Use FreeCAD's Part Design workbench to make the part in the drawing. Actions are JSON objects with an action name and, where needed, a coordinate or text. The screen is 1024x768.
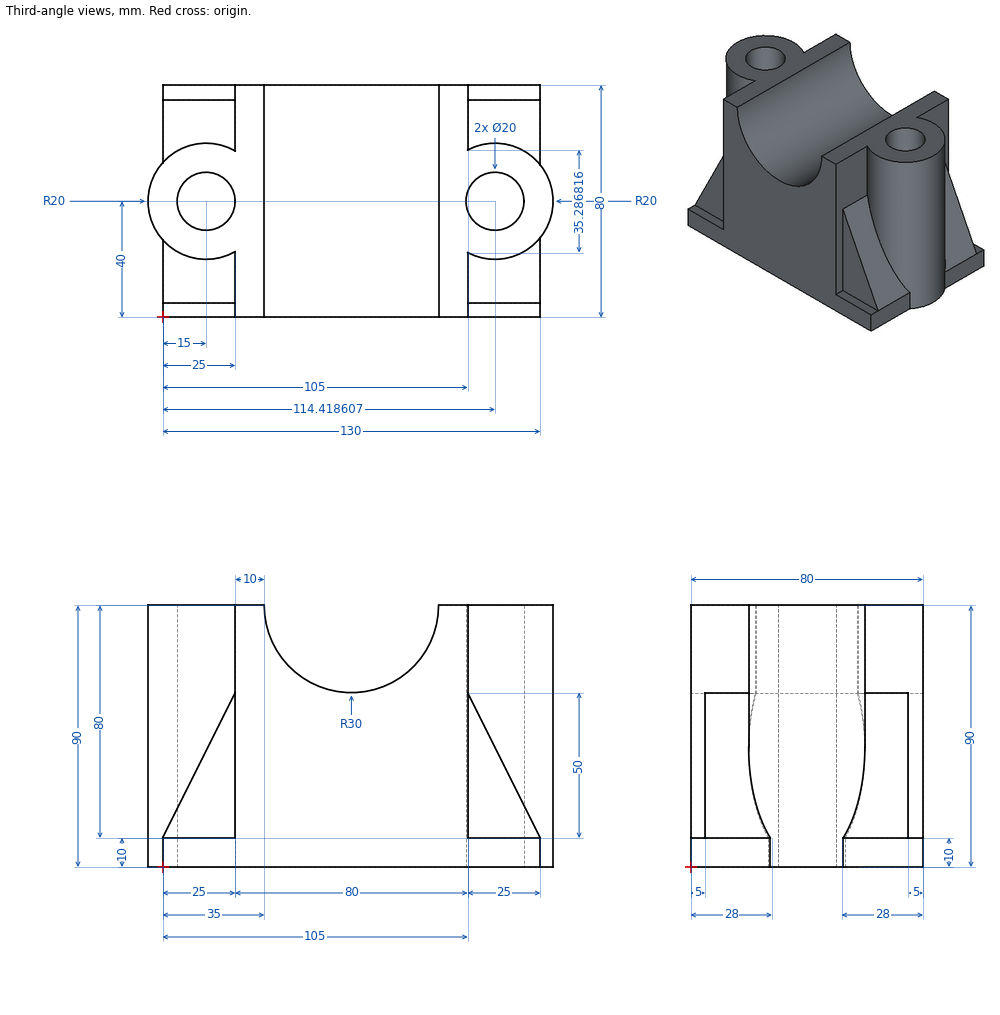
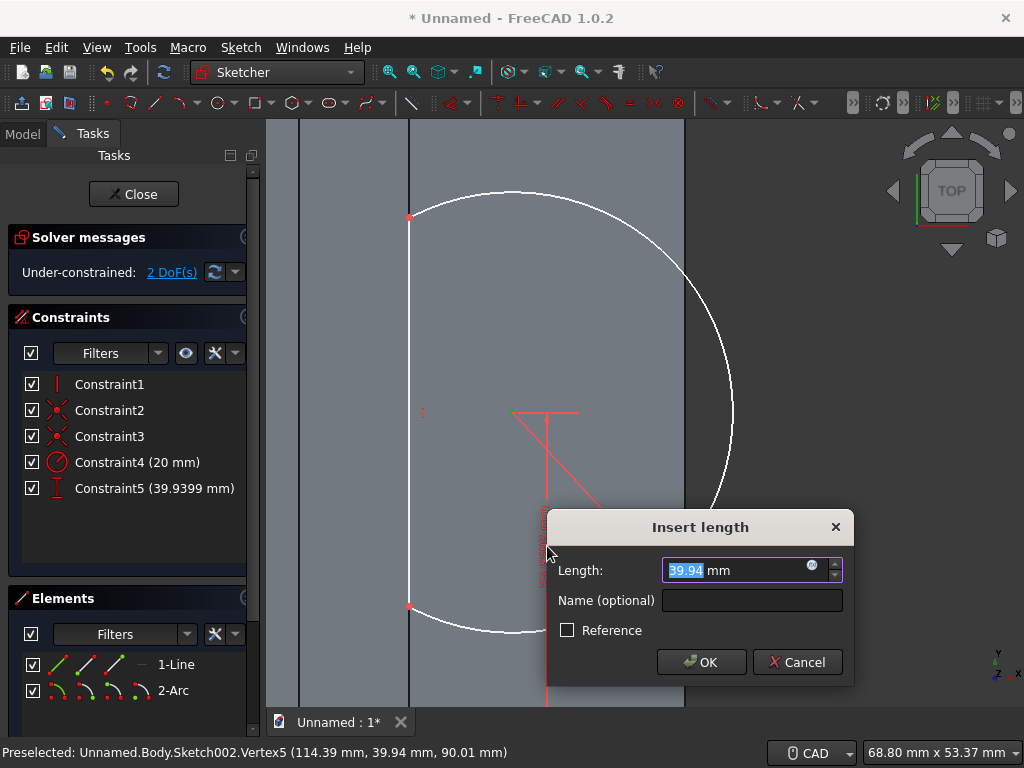
{"action": "type", "text": "40"}
{"action": "key", "text": "Return"}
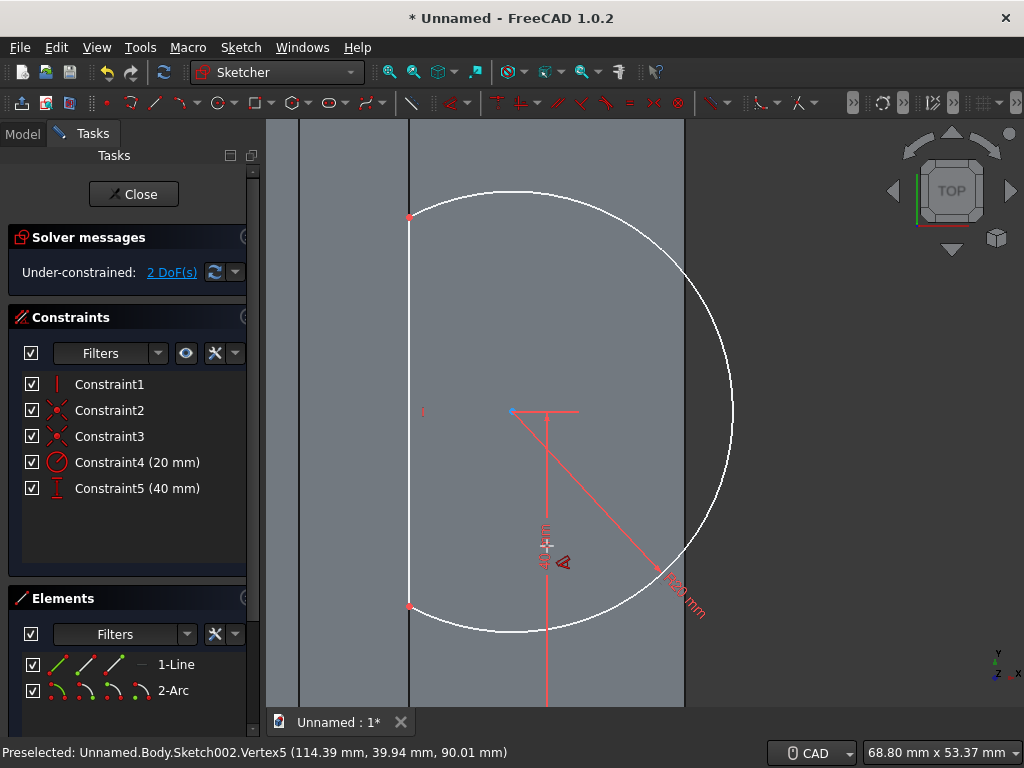
{"action": "left_click", "coordinate": [409, 217]}
{"action": "left_click", "coordinate": [352, 183]}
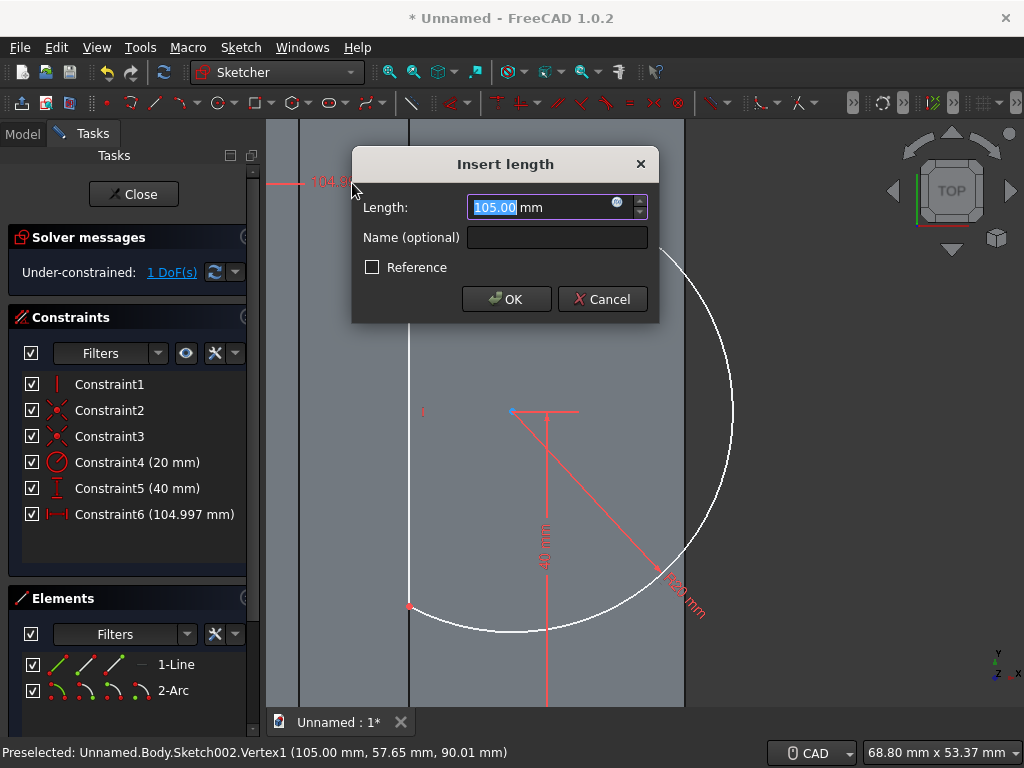
{"action": "type", "text": "105"}
{"action": "key", "text": "Return"}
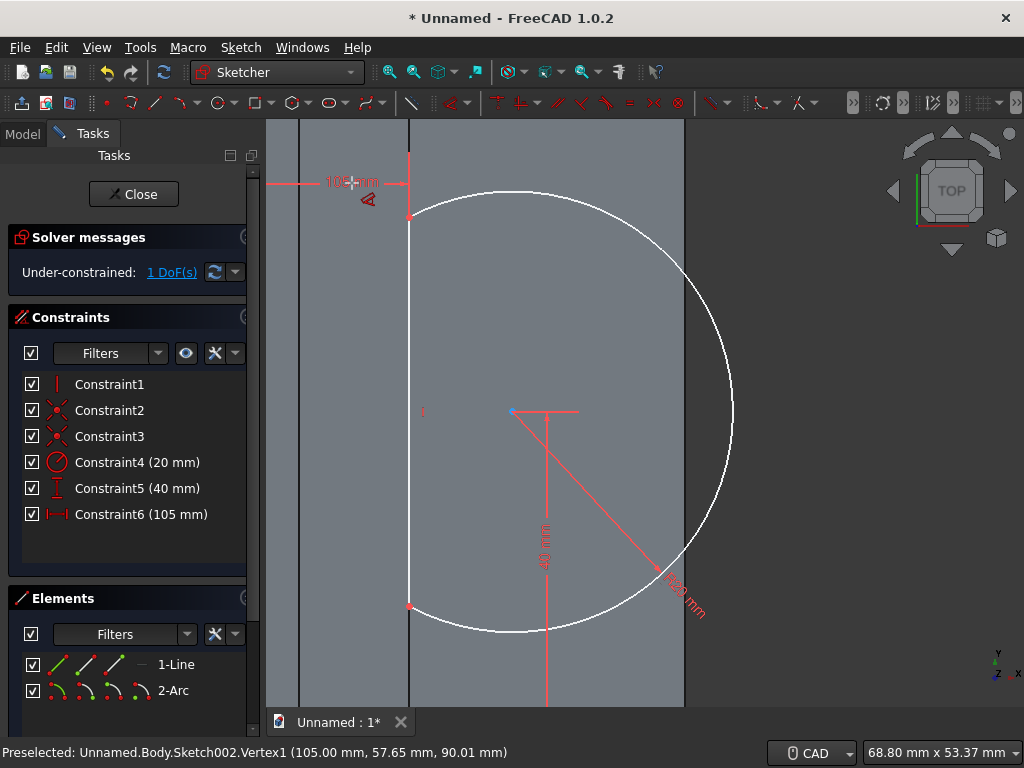
{"action": "left_click", "coordinate": [409, 334]}
{"action": "left_click", "coordinate": [375, 412]}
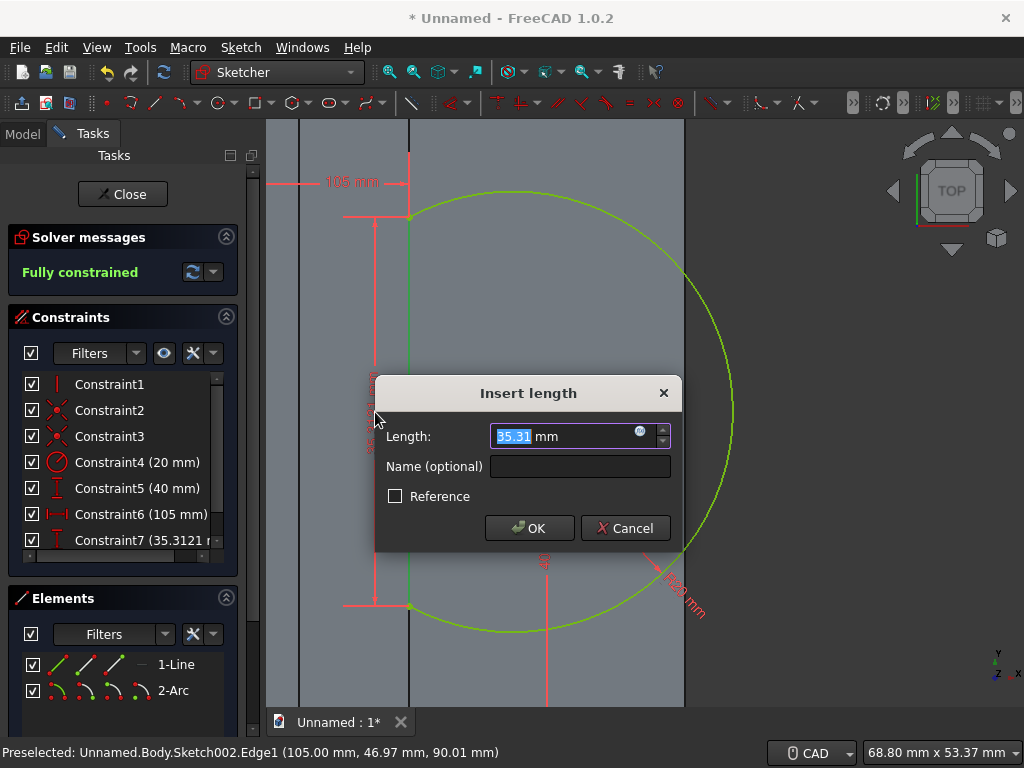
{"action": "type", "text": "35.286816"}
{"action": "key", "text": "Return"}
{"action": "key", "text": "Escape"}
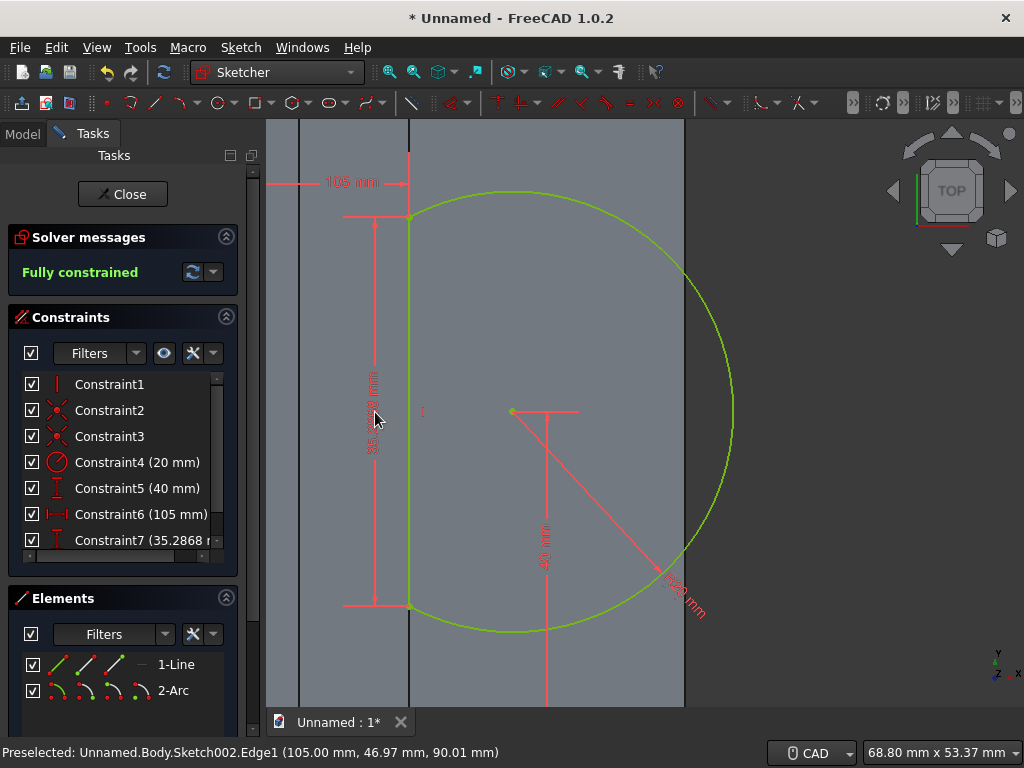
{"action": "left_click", "coordinate": [123, 194]}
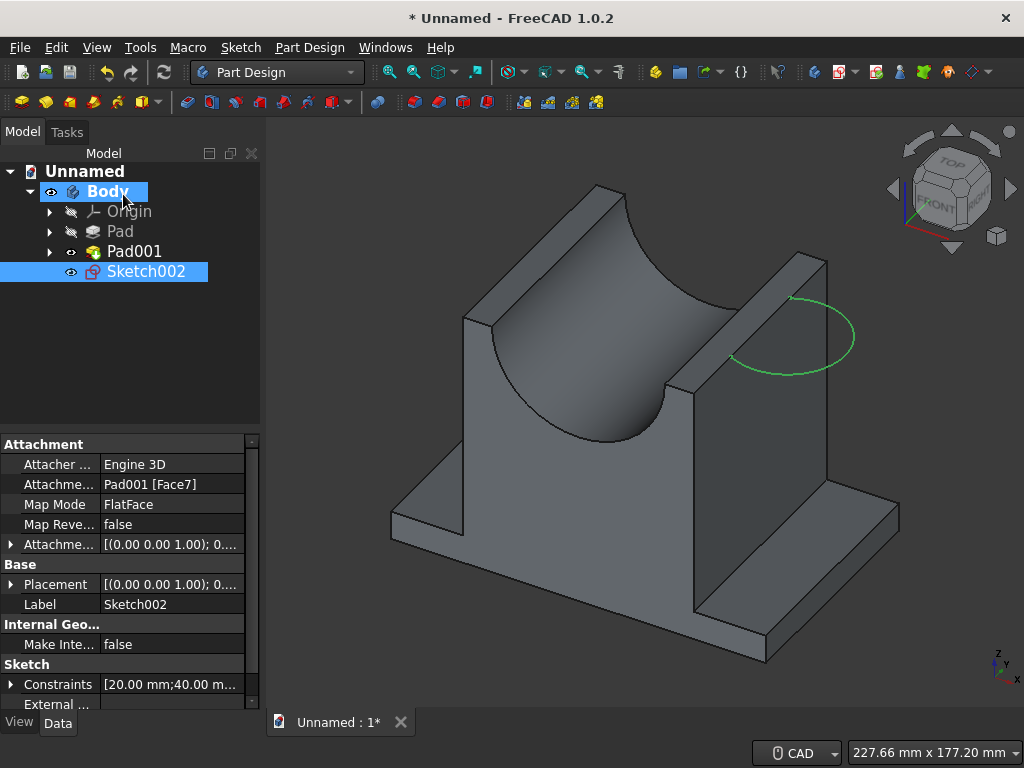
{"action": "left_click", "coordinate": [22, 102]}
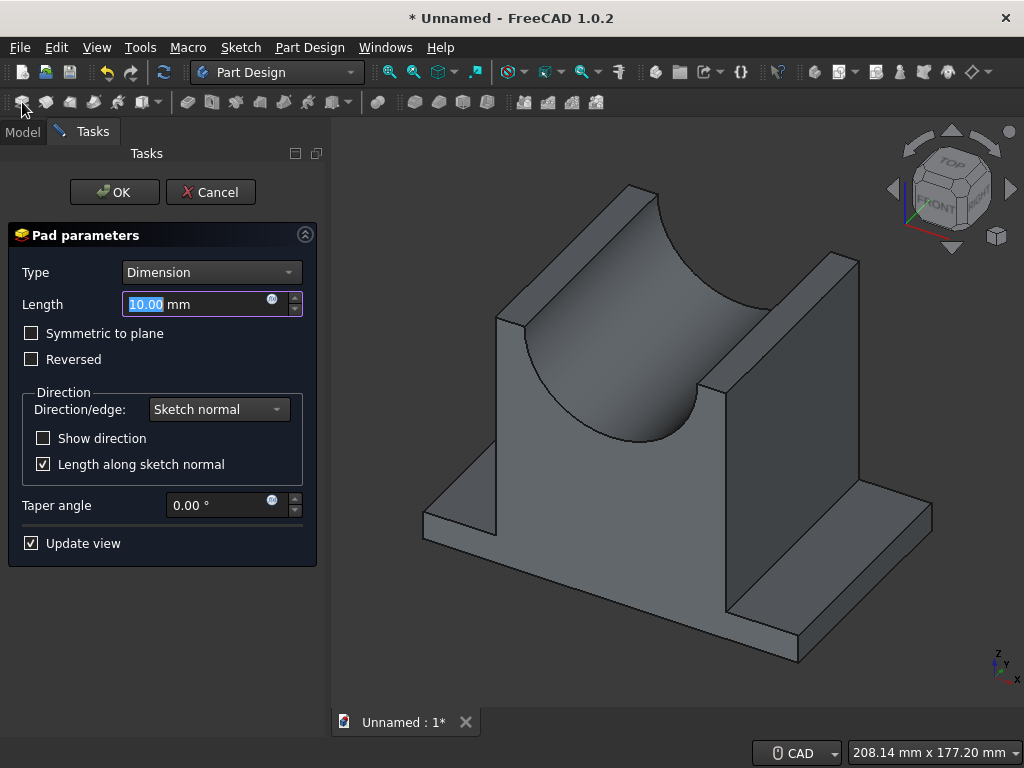
{"action": "type", "text": "90"}
{"action": "key", "text": "Tab"}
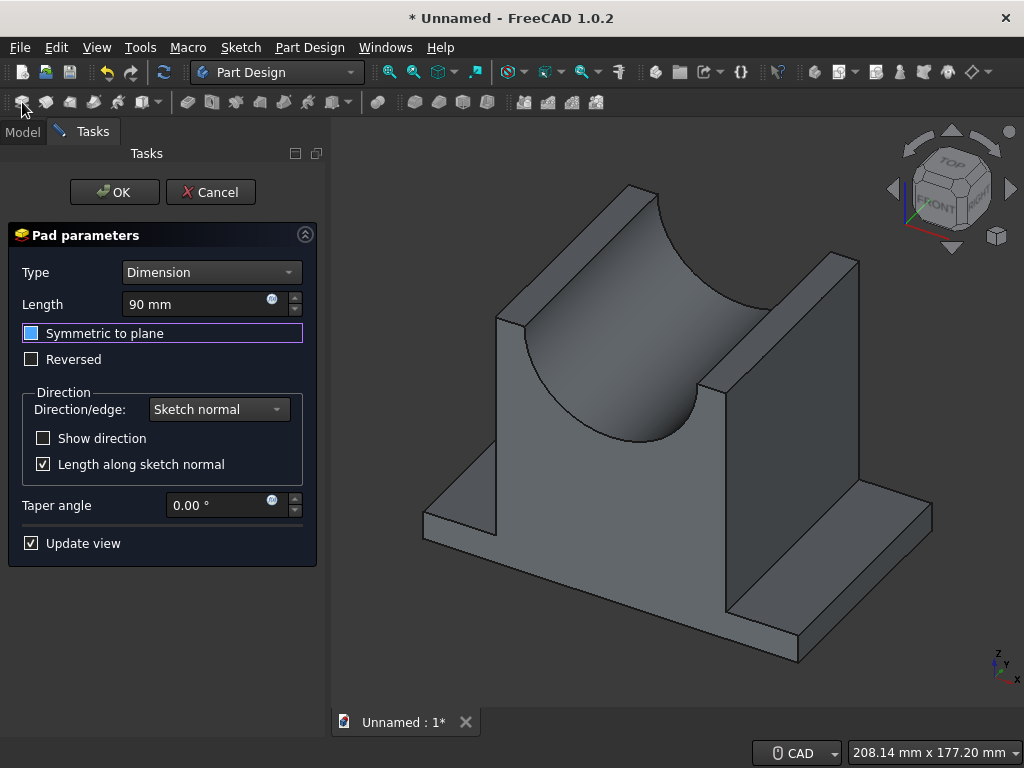
{"action": "left_click", "coordinate": [30, 359]}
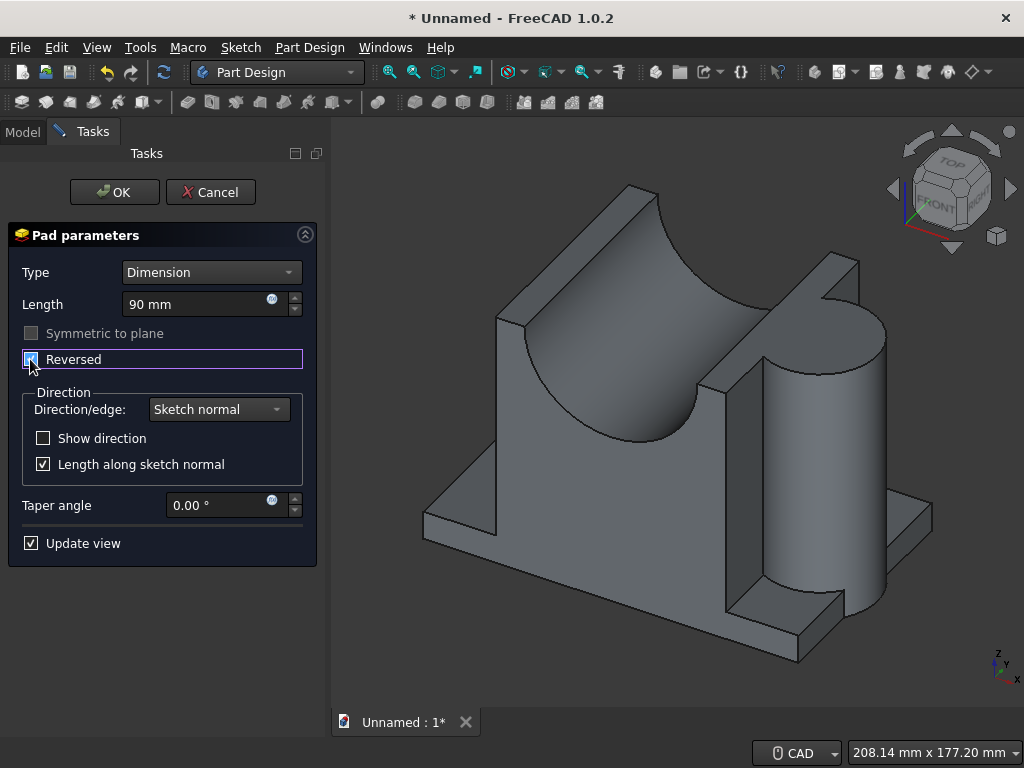
{"action": "left_click", "coordinate": [115, 192]}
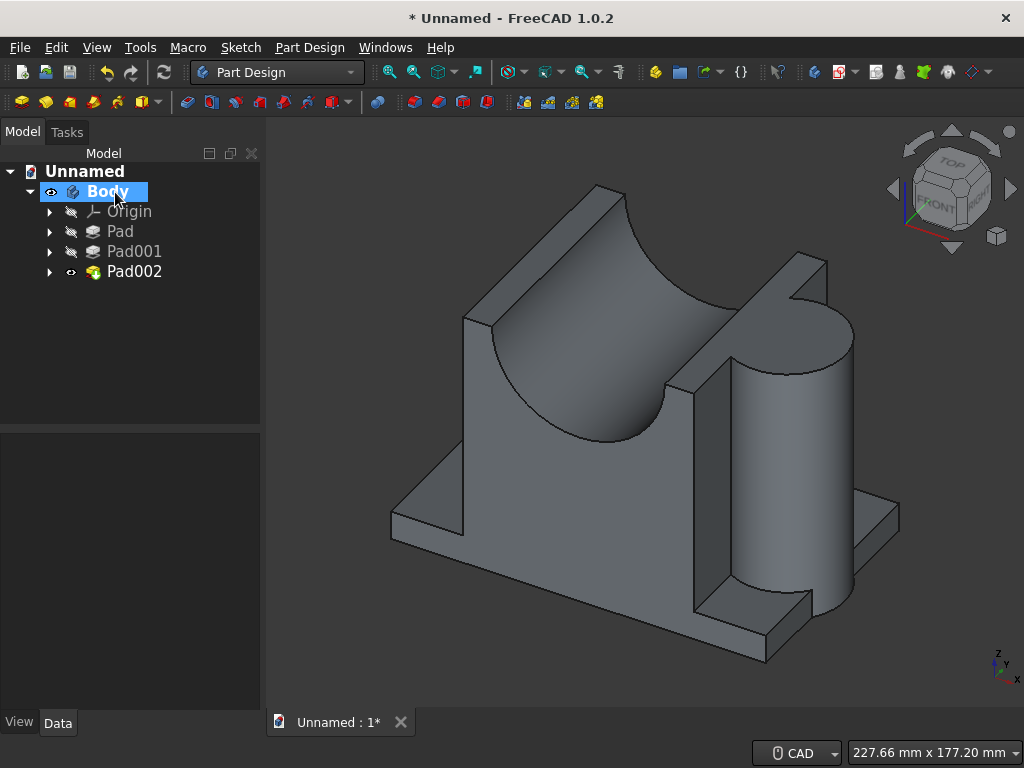
{"action": "left_click", "coordinate": [788, 336]}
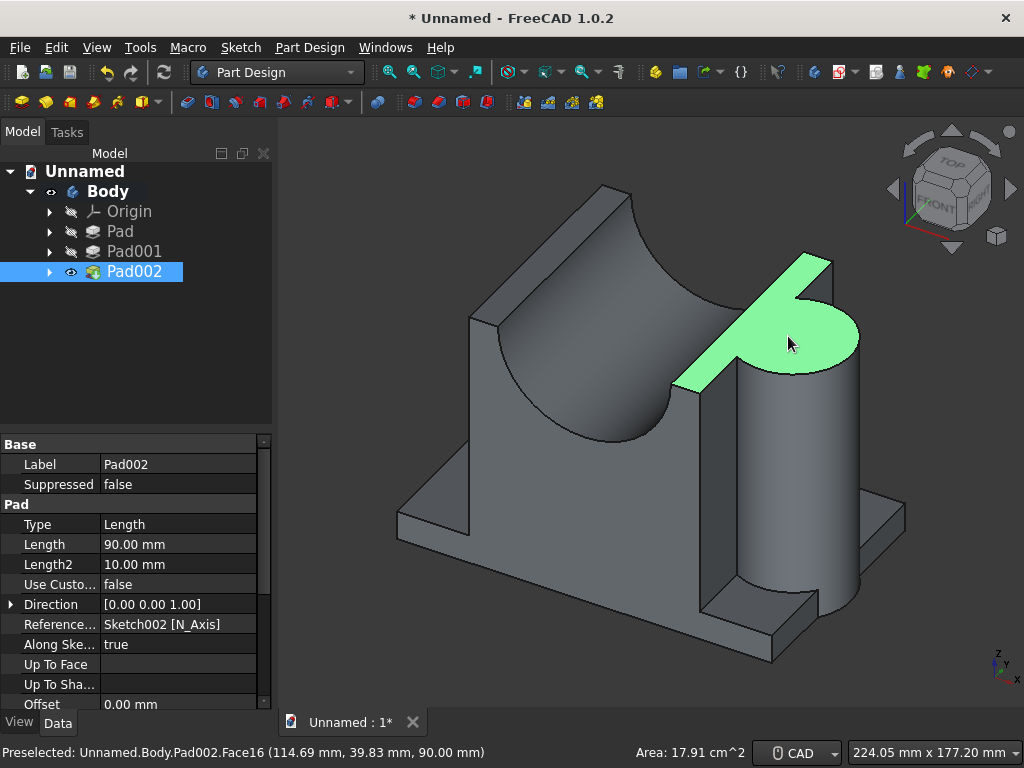
{"action": "left_click", "coordinate": [840, 72]}